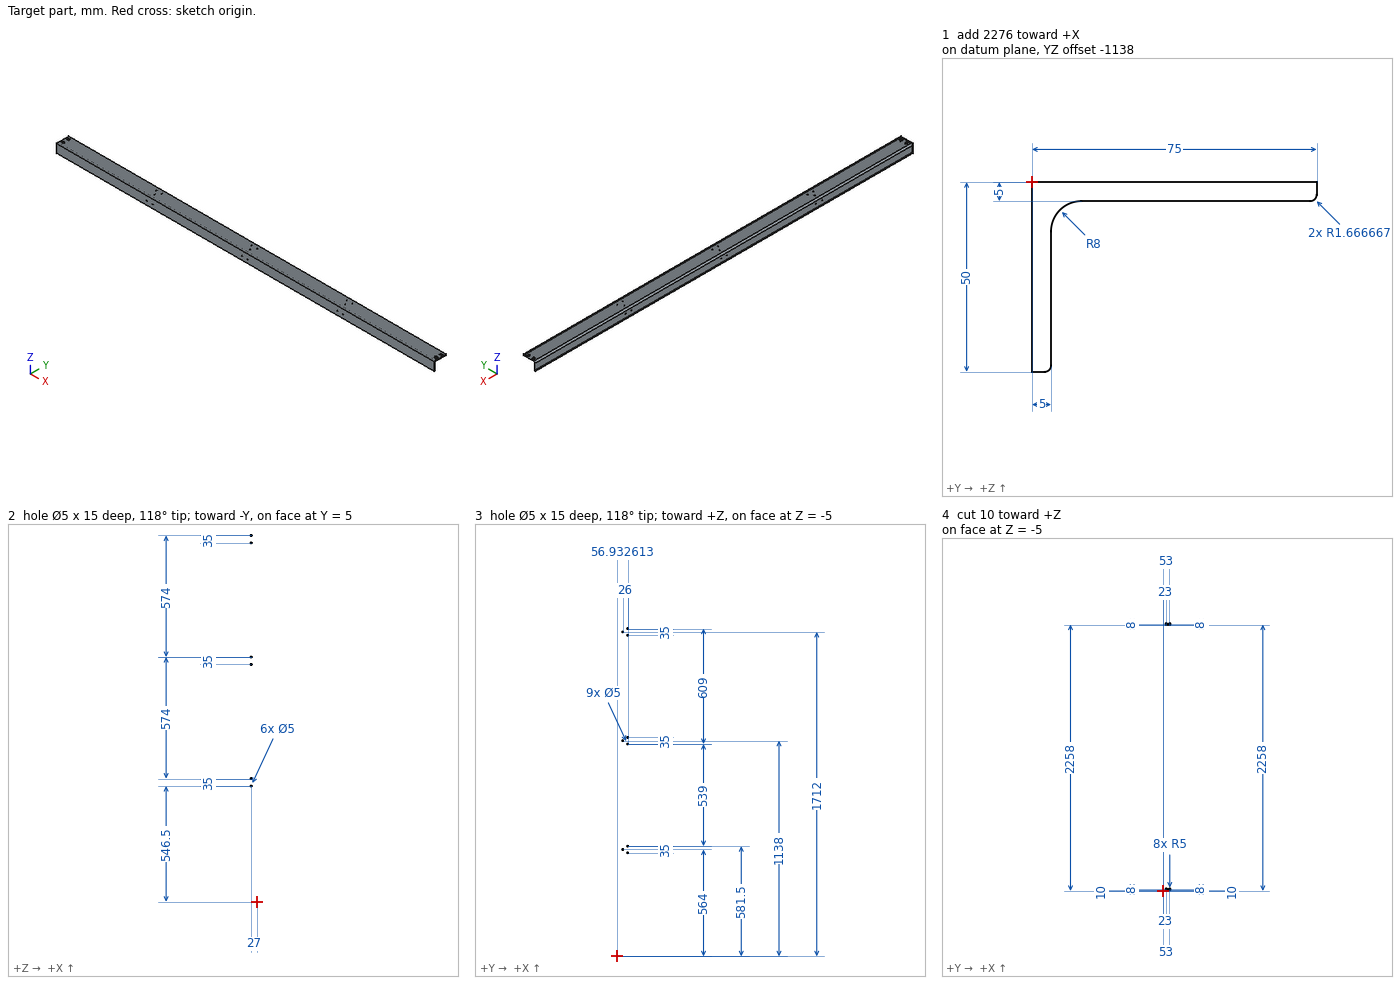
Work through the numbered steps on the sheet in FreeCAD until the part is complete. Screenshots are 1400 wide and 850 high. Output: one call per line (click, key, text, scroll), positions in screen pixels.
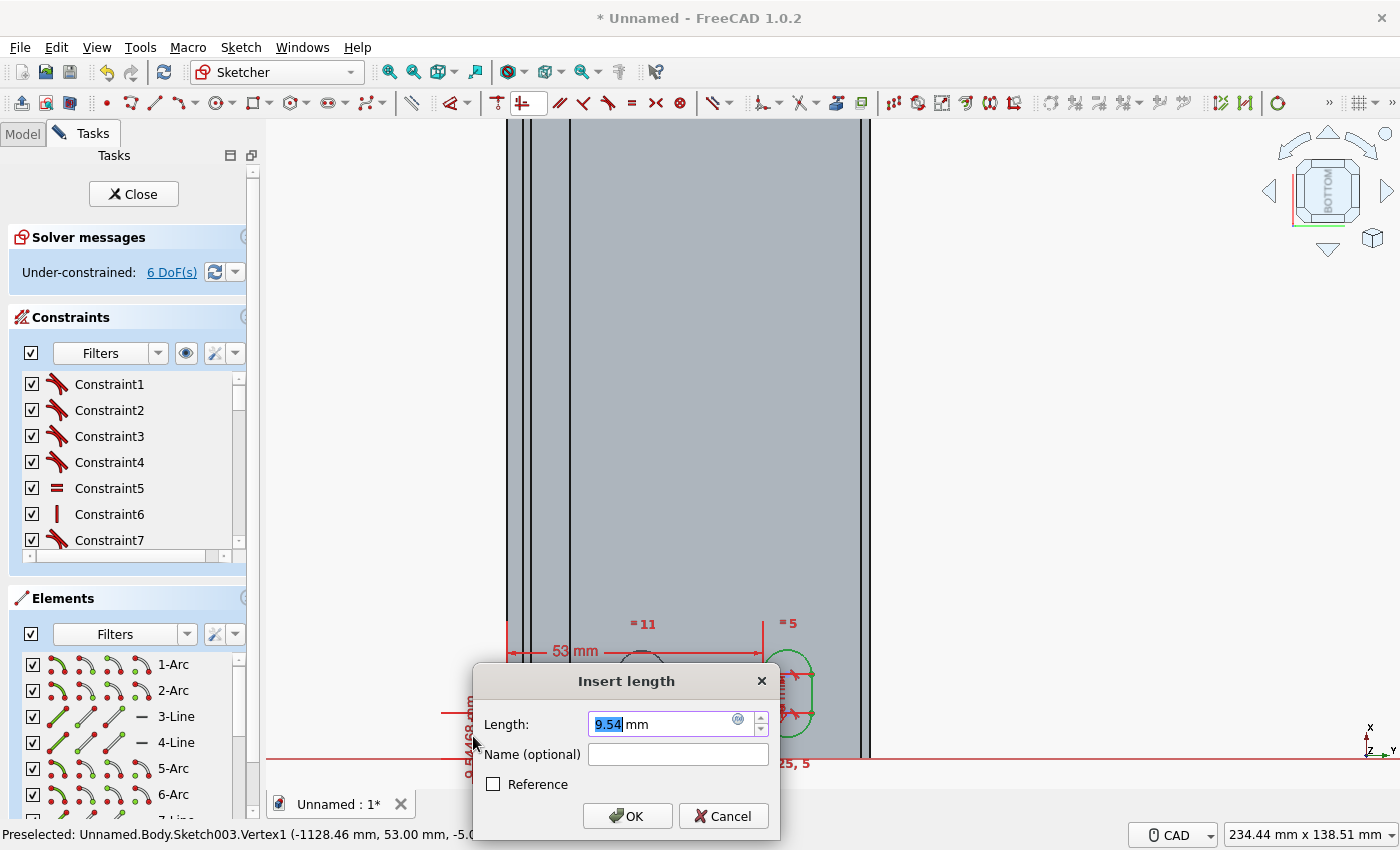
text(10)
key(Return)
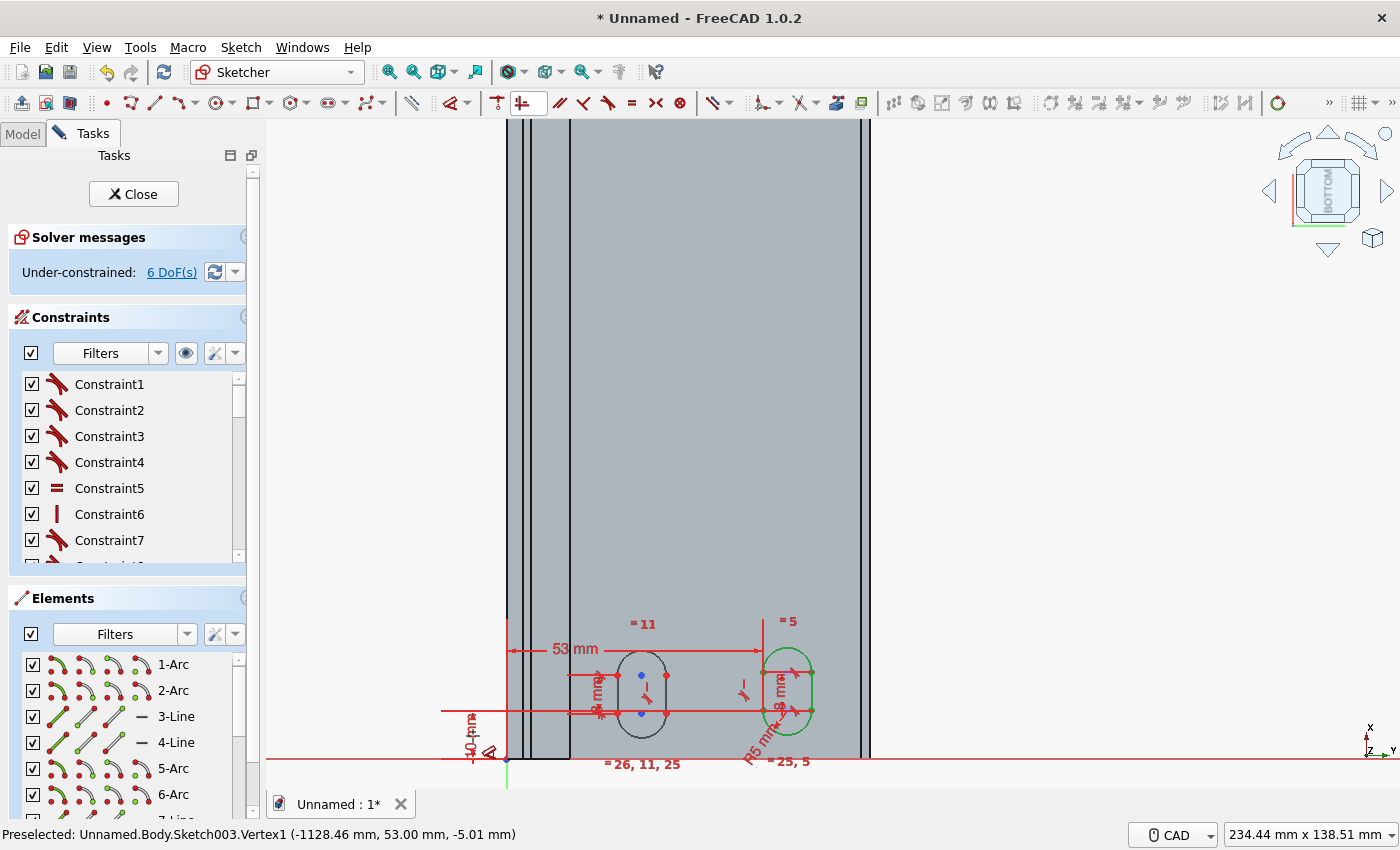
click(618, 714)
click(523, 680)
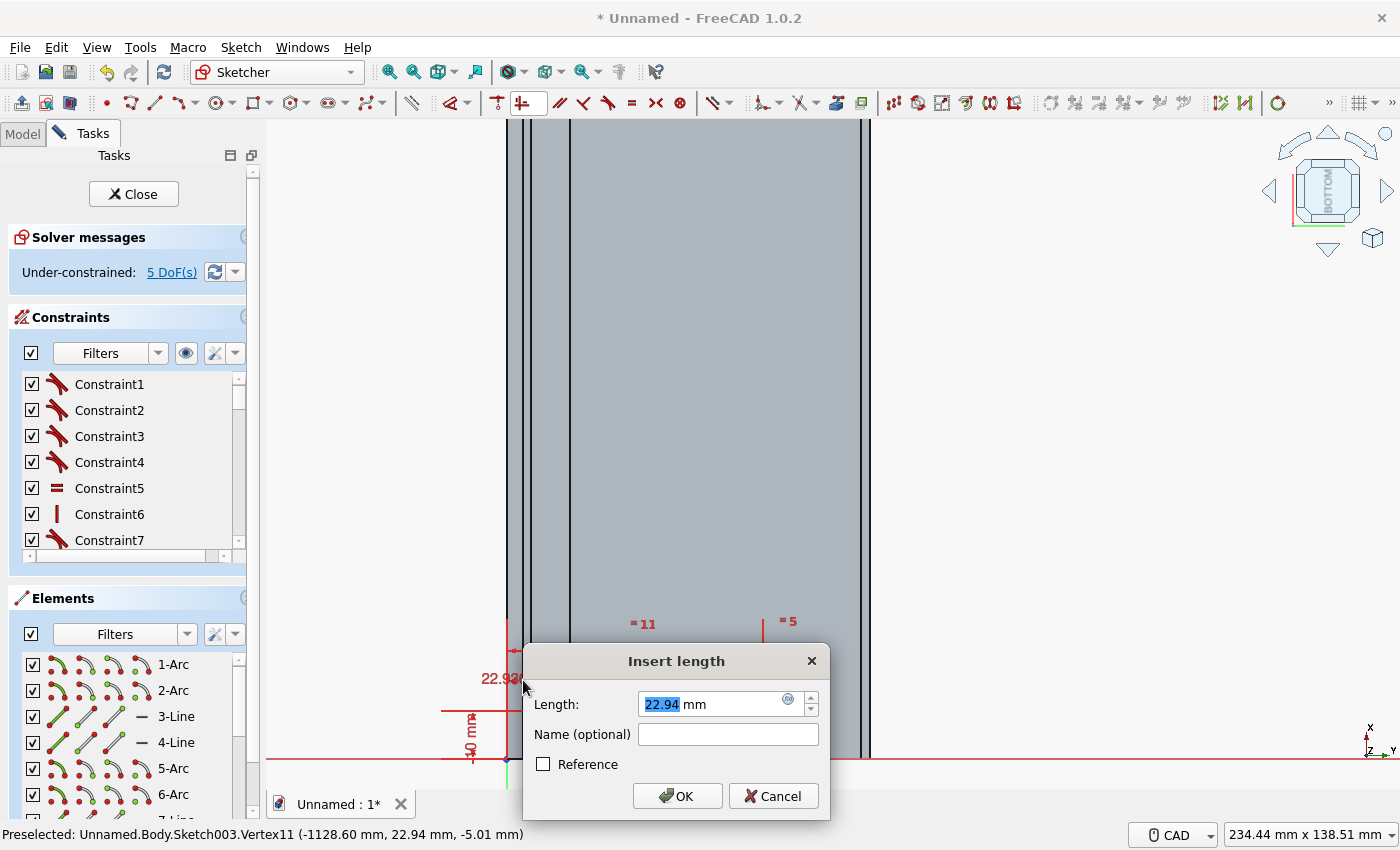
text(23)
key(Return)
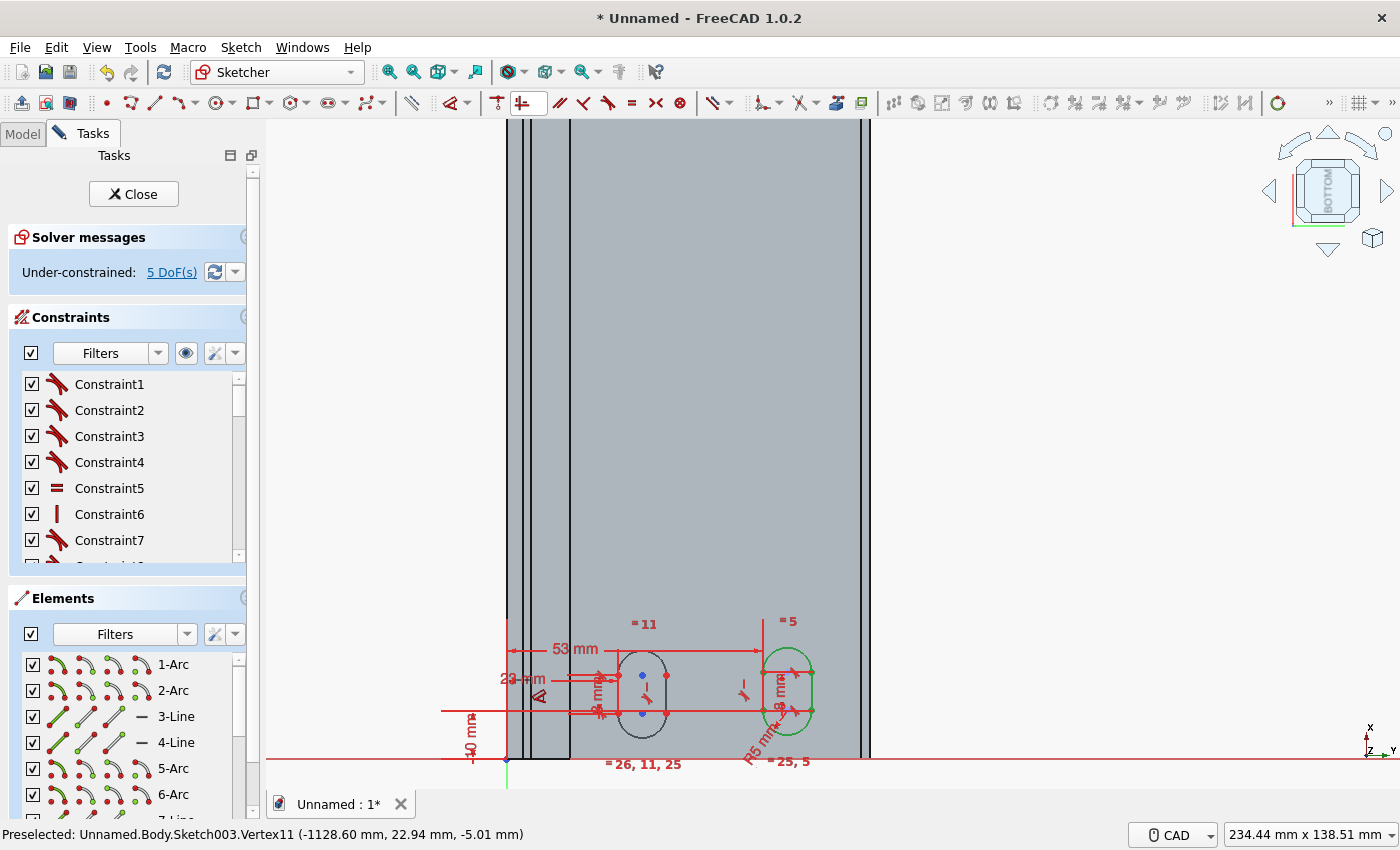
click(618, 714)
click(676, 736)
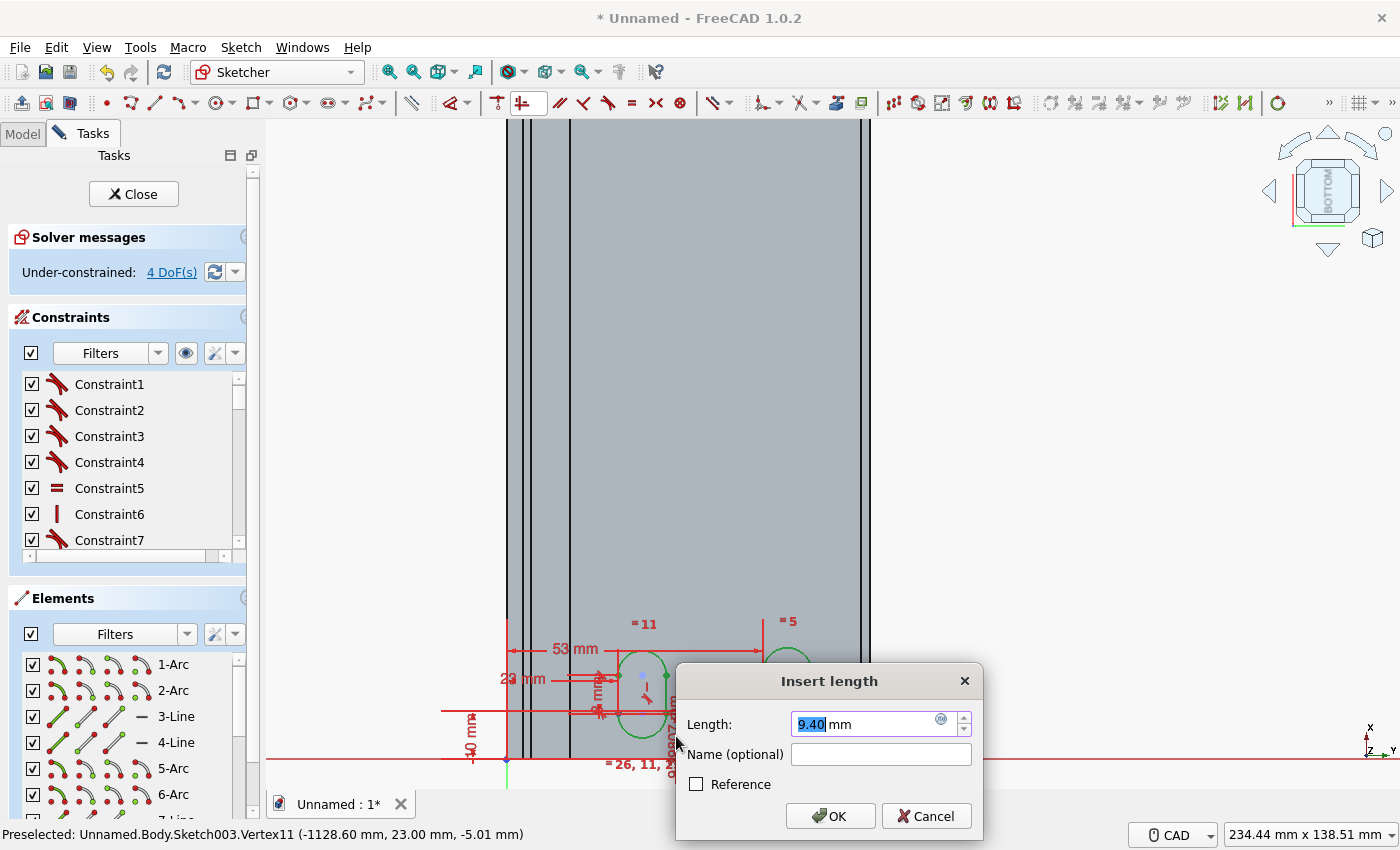
text(10)
key(Return)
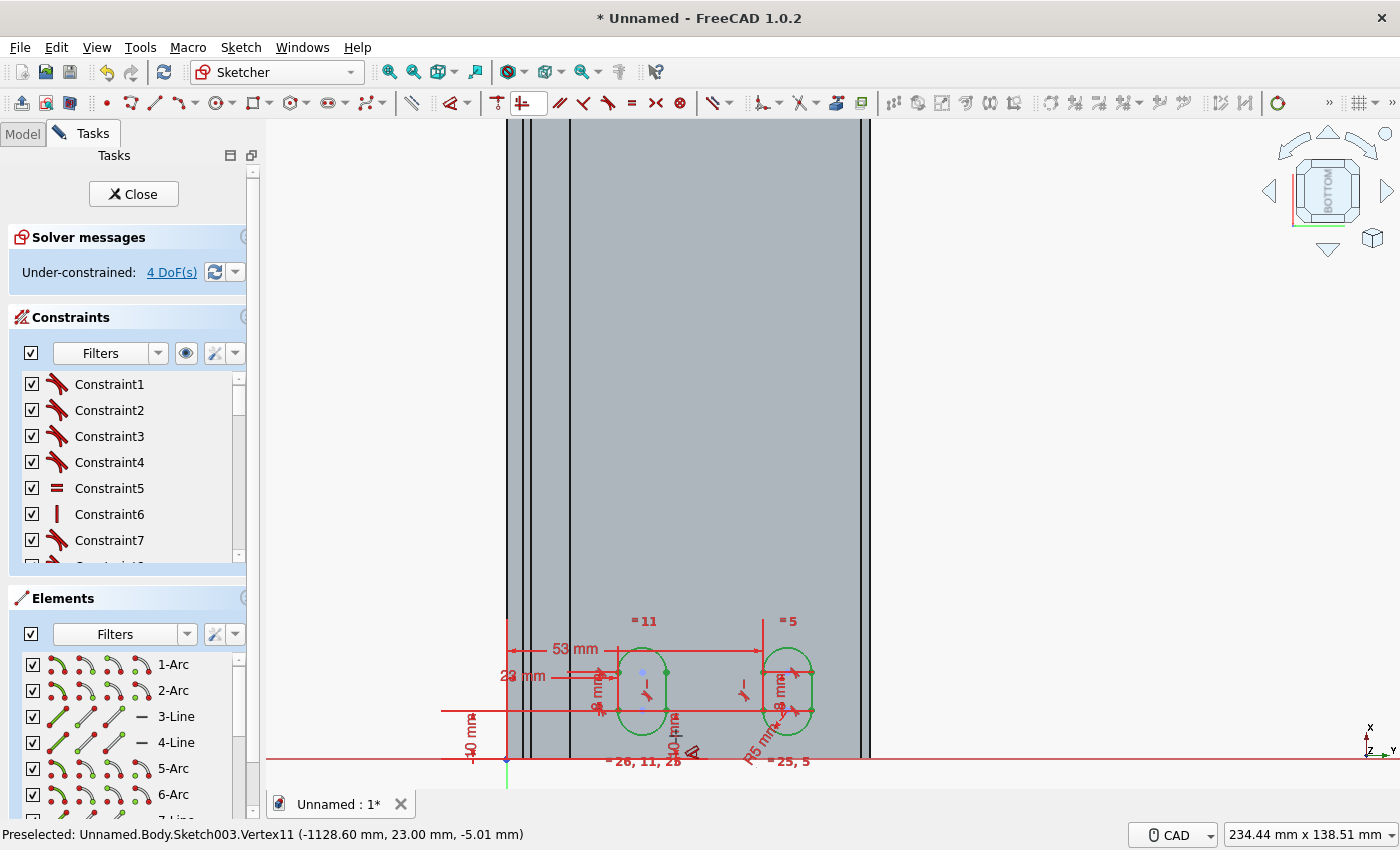
scroll(770, 726, down, 15)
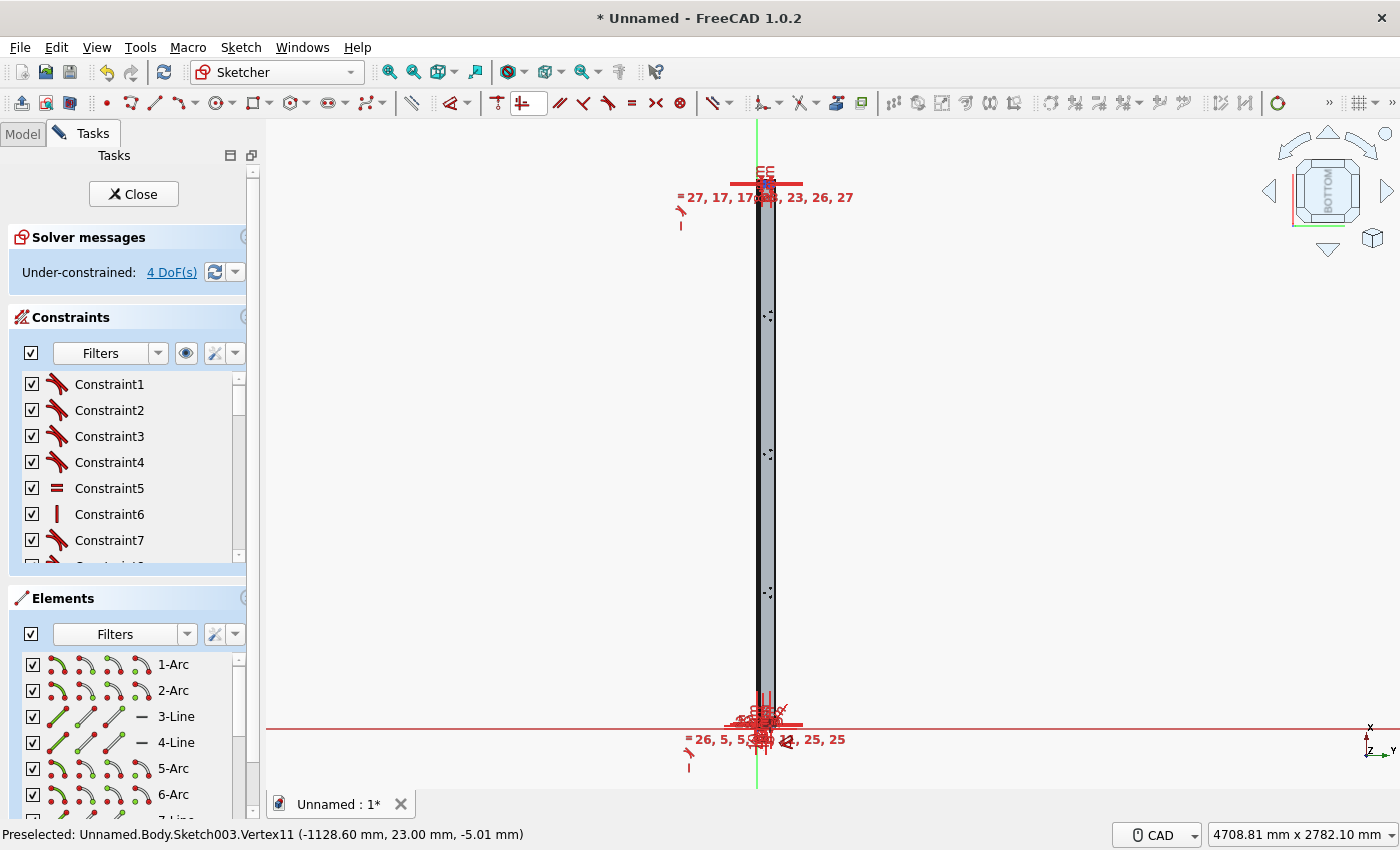
scroll(770, 185, up, 12)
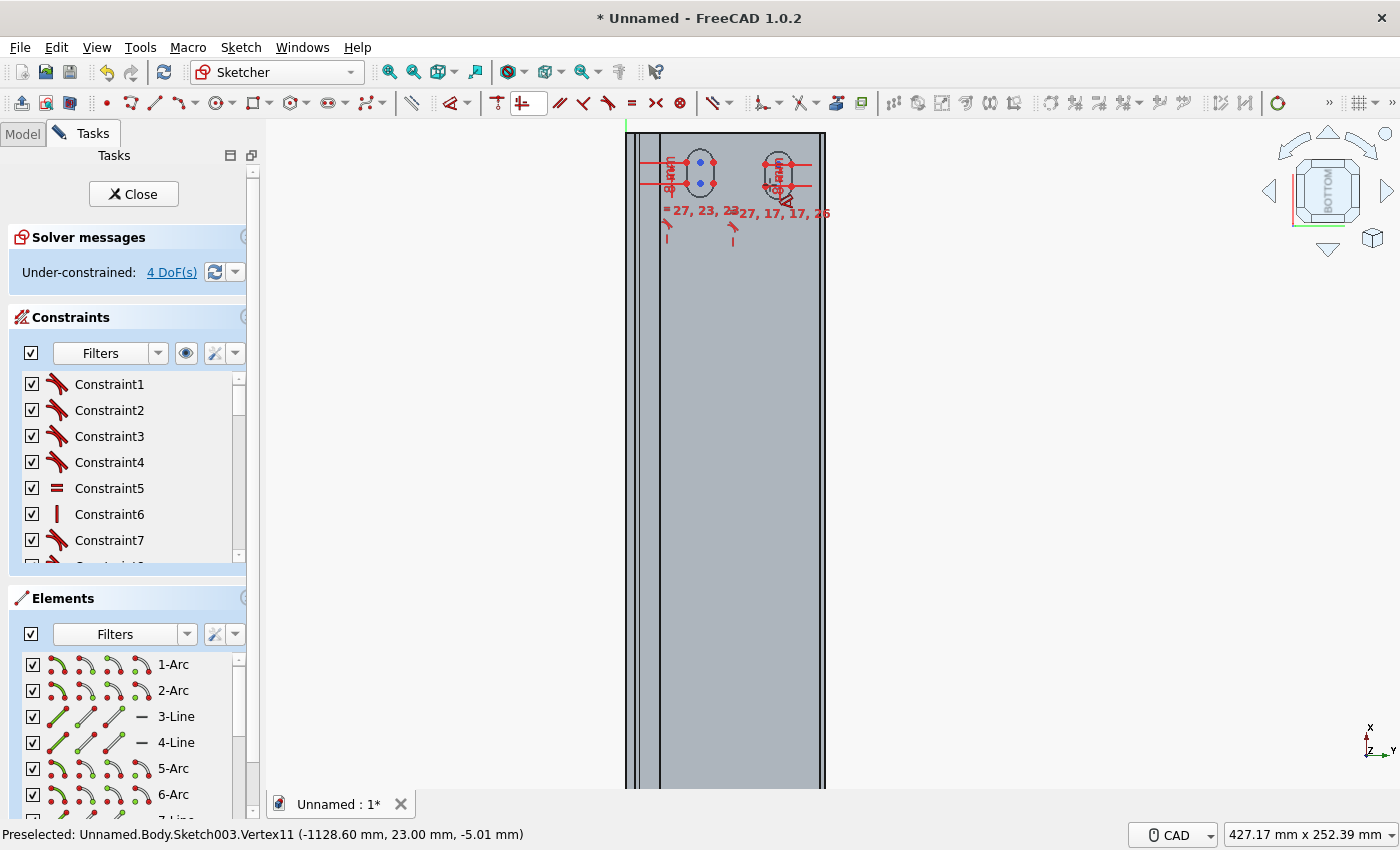
click(765, 186)
click(663, 152)